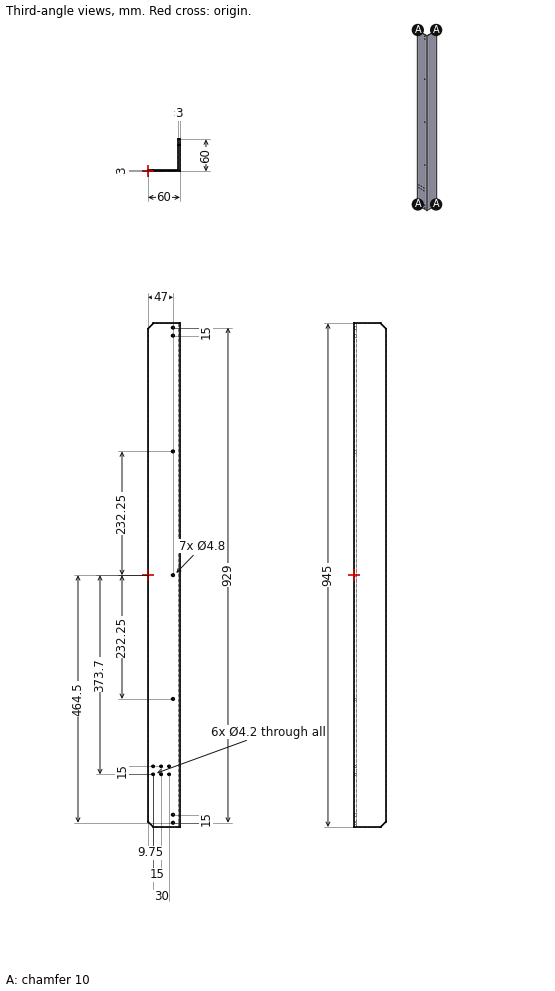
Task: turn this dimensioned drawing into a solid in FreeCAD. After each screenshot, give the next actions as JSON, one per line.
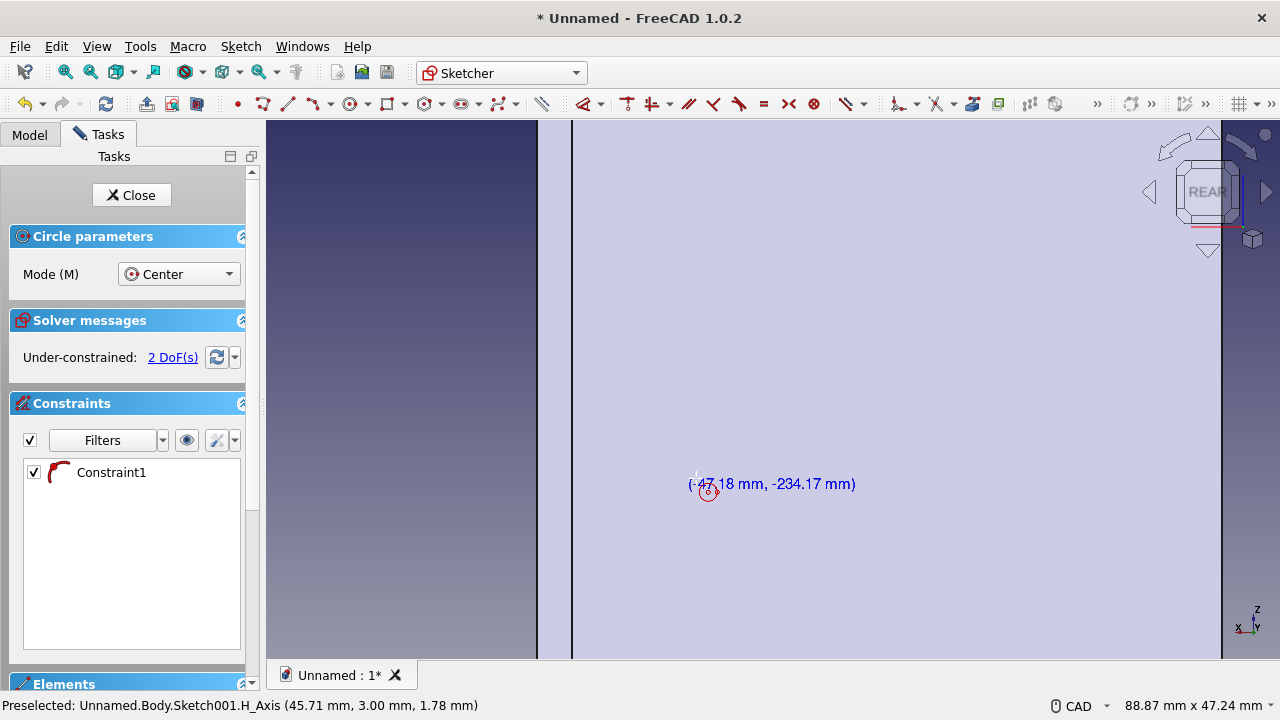
{"action": "scroll", "coordinate": [696, 478], "scroll_direction": "down", "scroll_amount": 17}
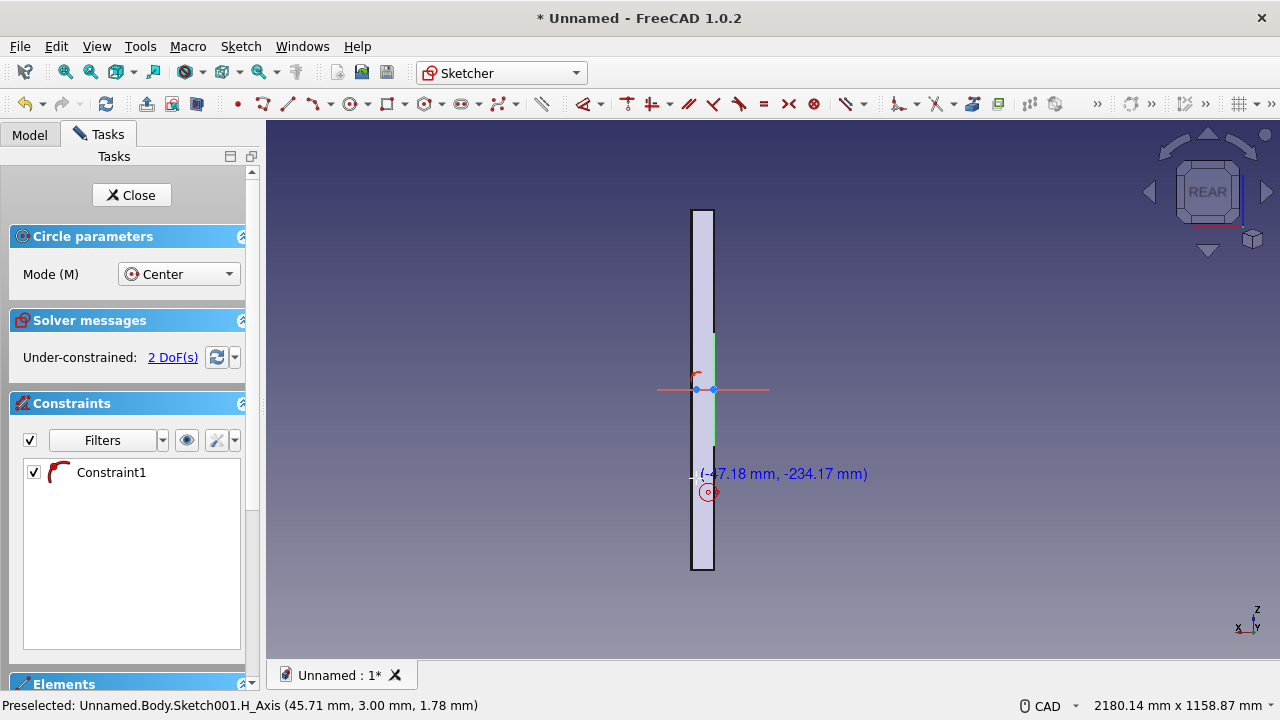
{"action": "left_click", "coordinate": [696, 478]}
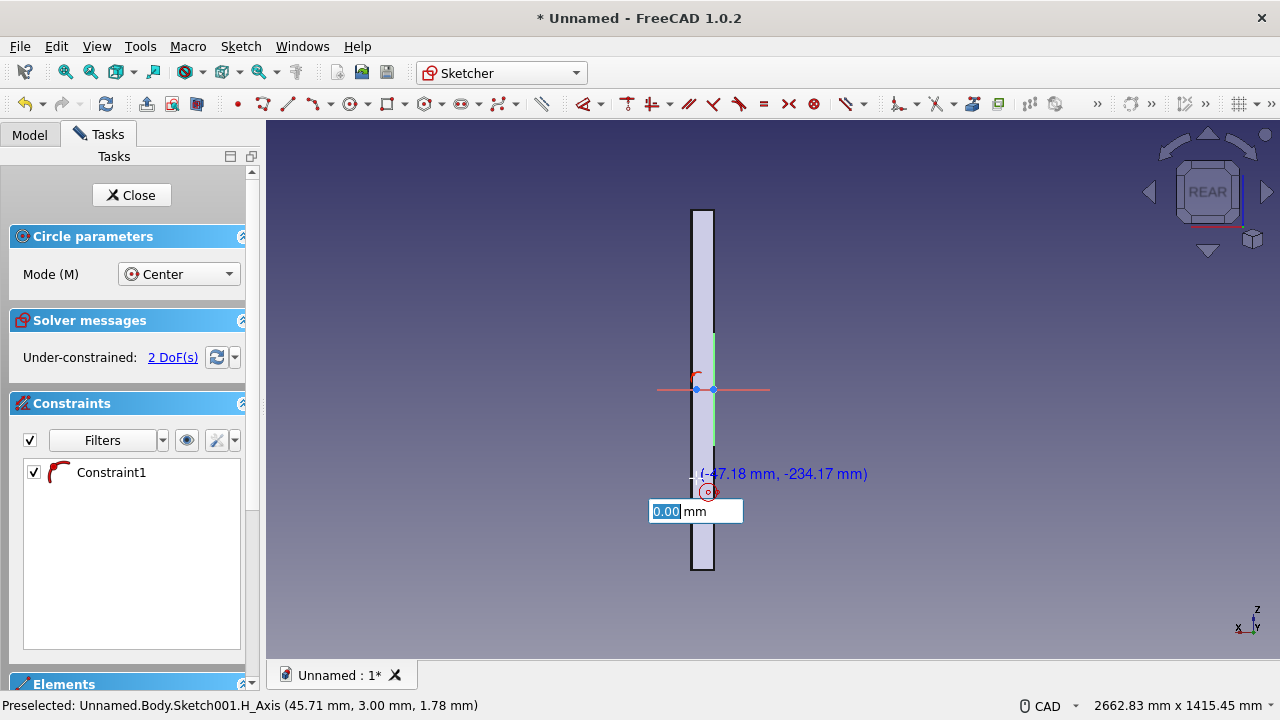
{"action": "scroll", "coordinate": [697, 478], "scroll_direction": "up", "scroll_amount": 15}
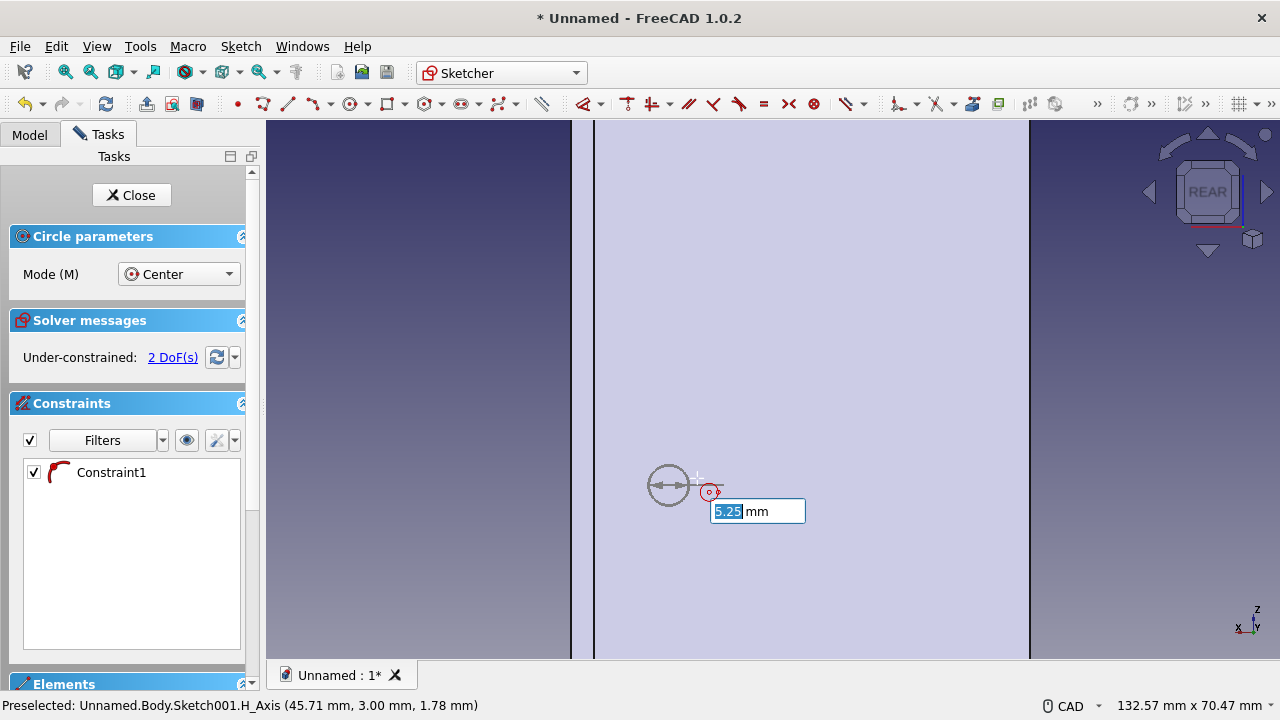
{"action": "left_click", "coordinate": [683, 458]}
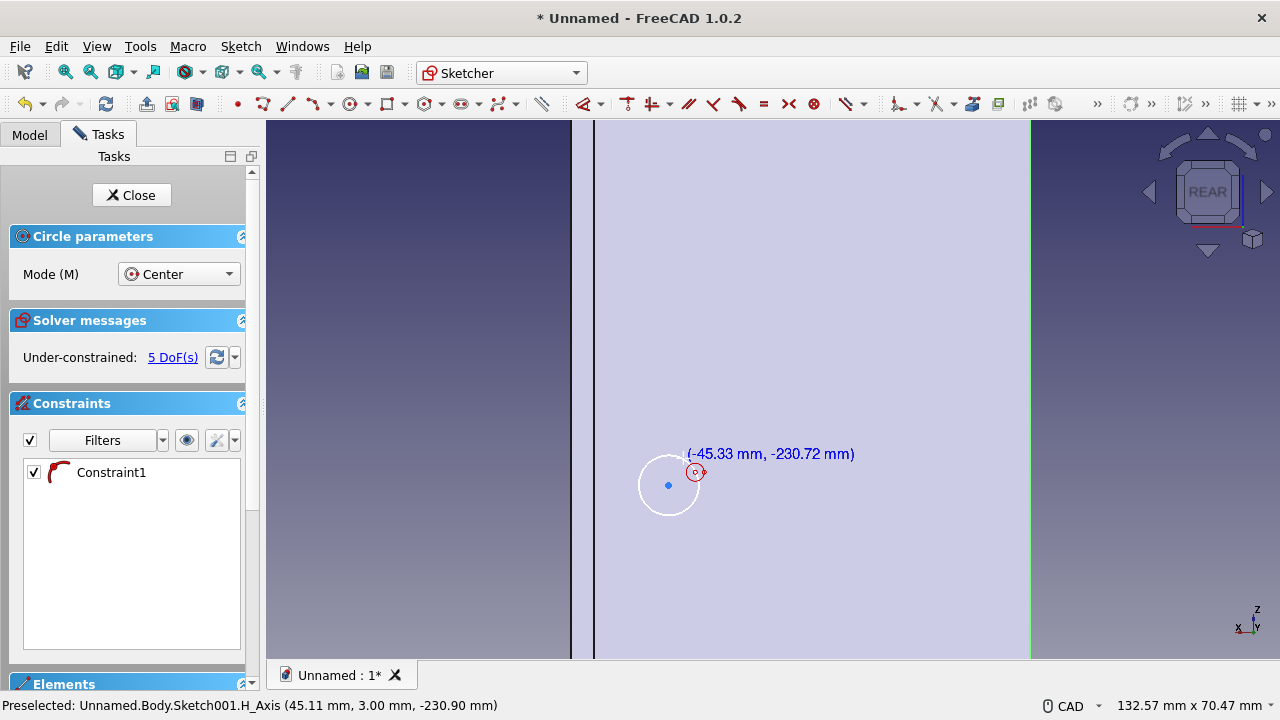
{"action": "scroll", "coordinate": [697, 478], "scroll_direction": "down", "scroll_amount": 15}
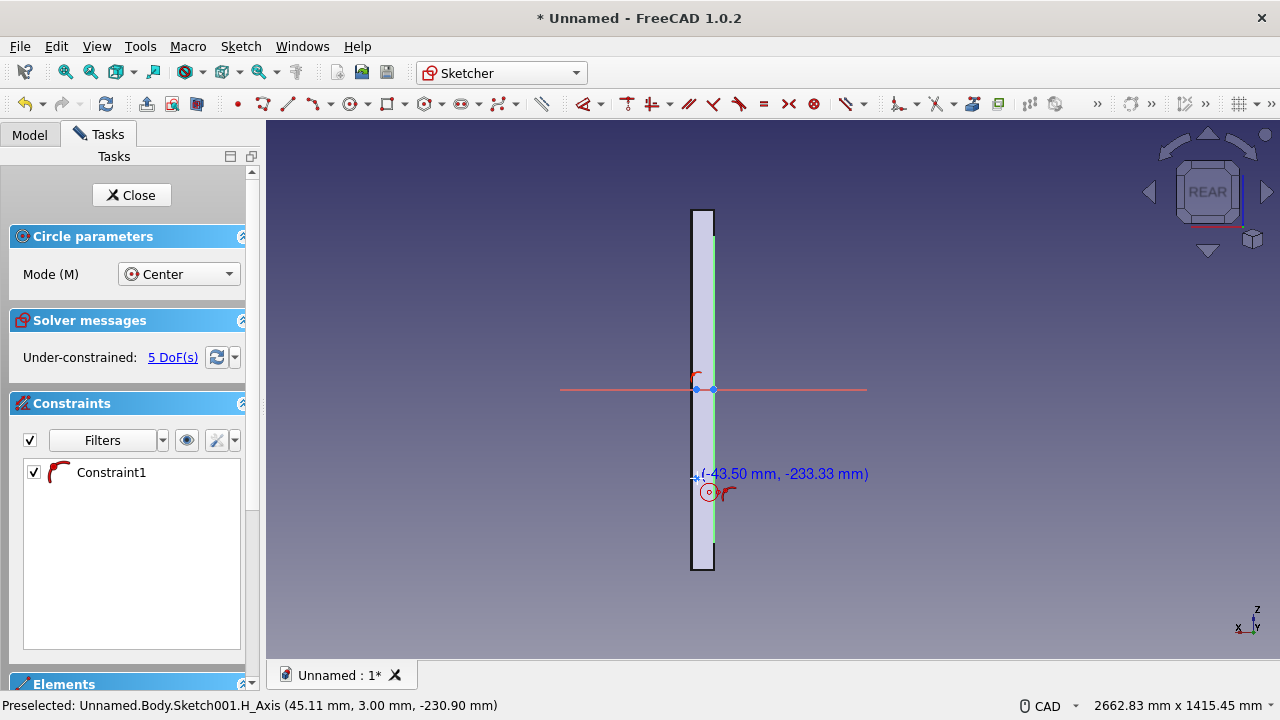
{"action": "scroll", "coordinate": [696, 567], "scroll_direction": "up", "scroll_amount": 17}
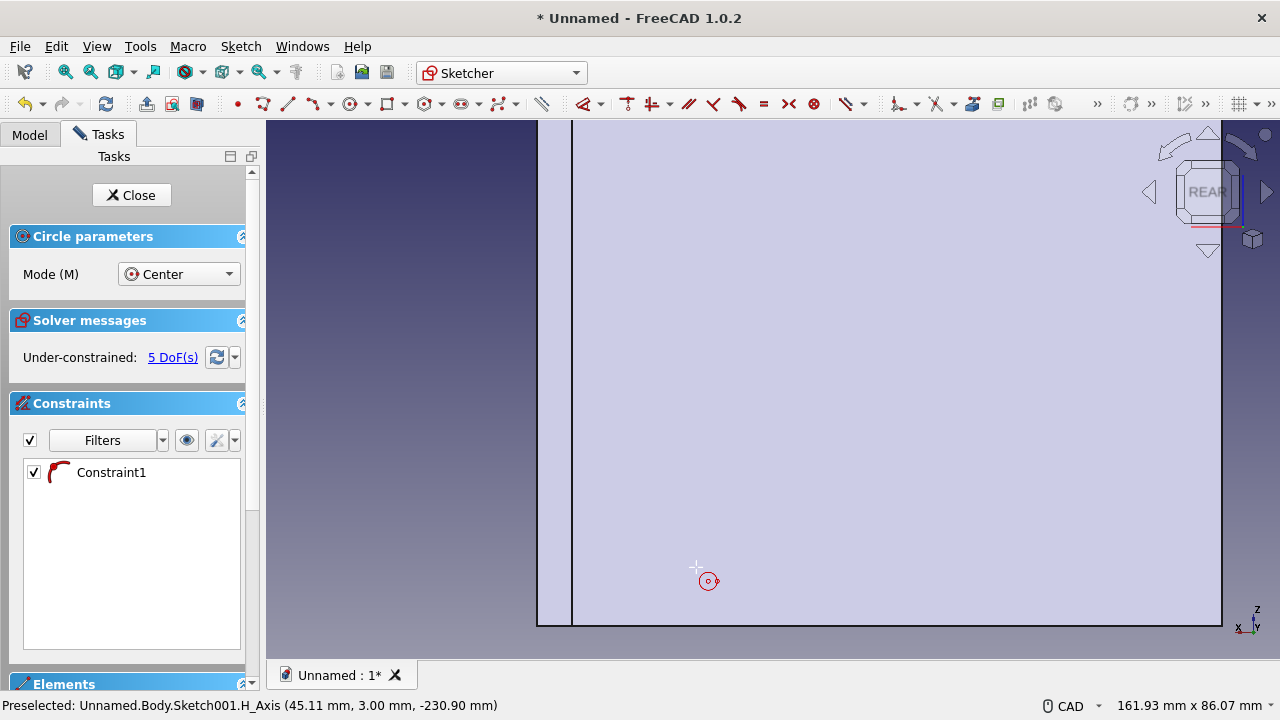
{"action": "scroll", "coordinate": [696, 567], "scroll_direction": "down", "scroll_amount": 17}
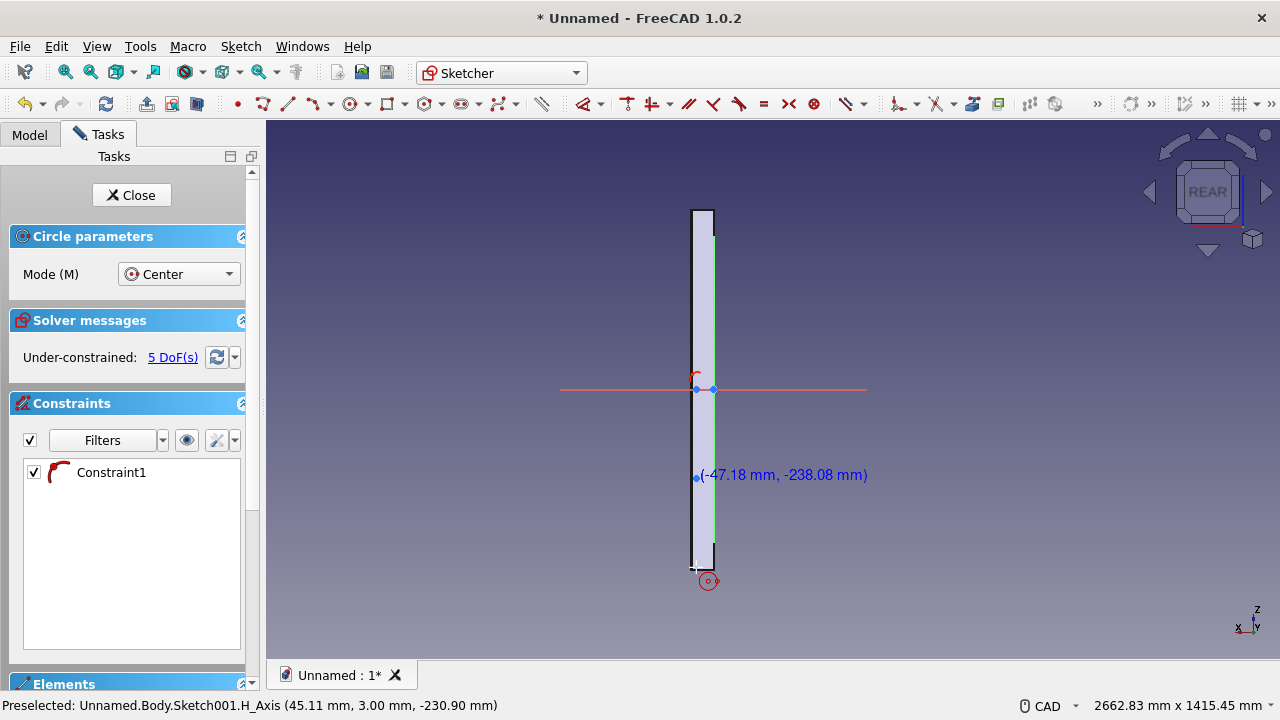
{"action": "left_click", "coordinate": [696, 567]}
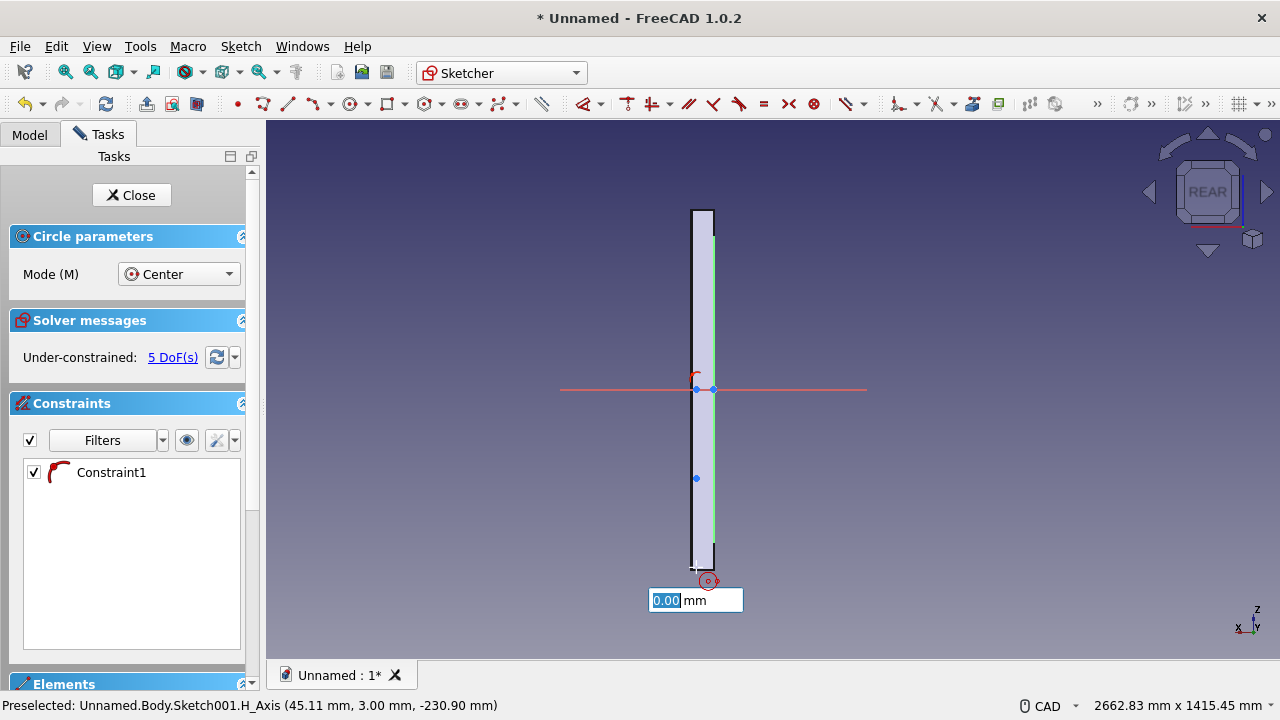
{"action": "scroll", "coordinate": [697, 566], "scroll_direction": "up", "scroll_amount": 15}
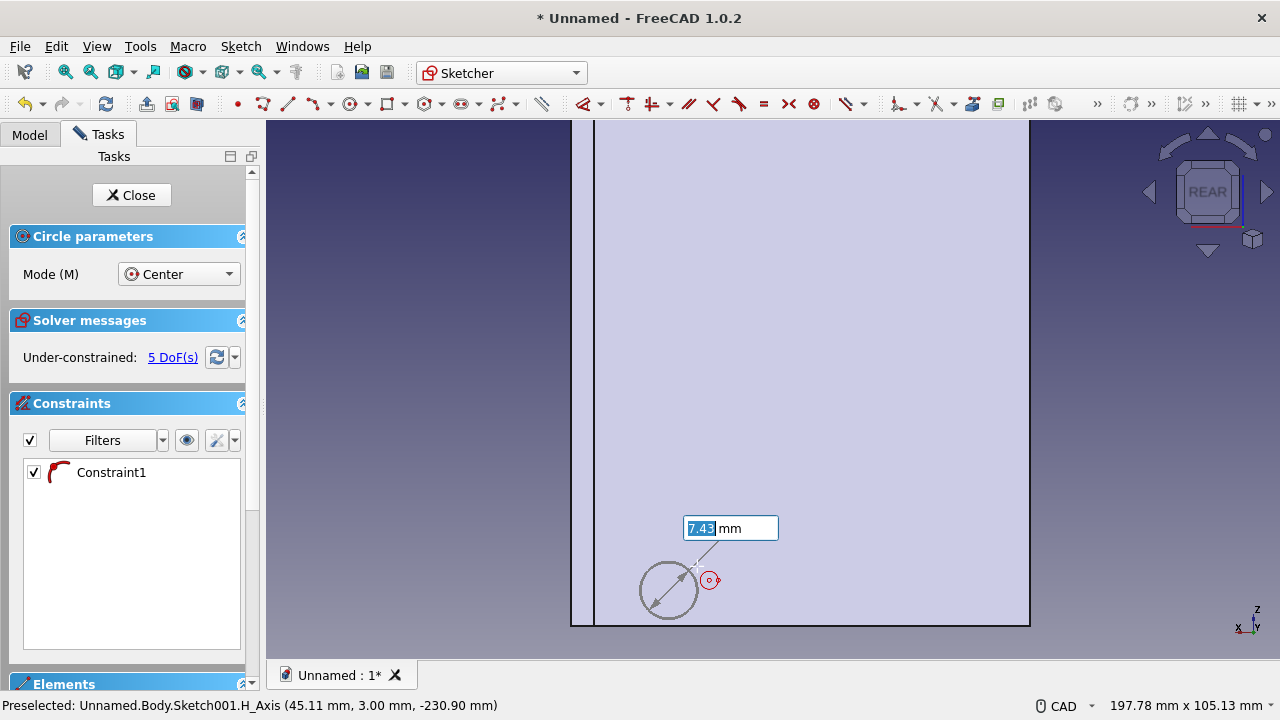
{"action": "left_click", "coordinate": [683, 551]}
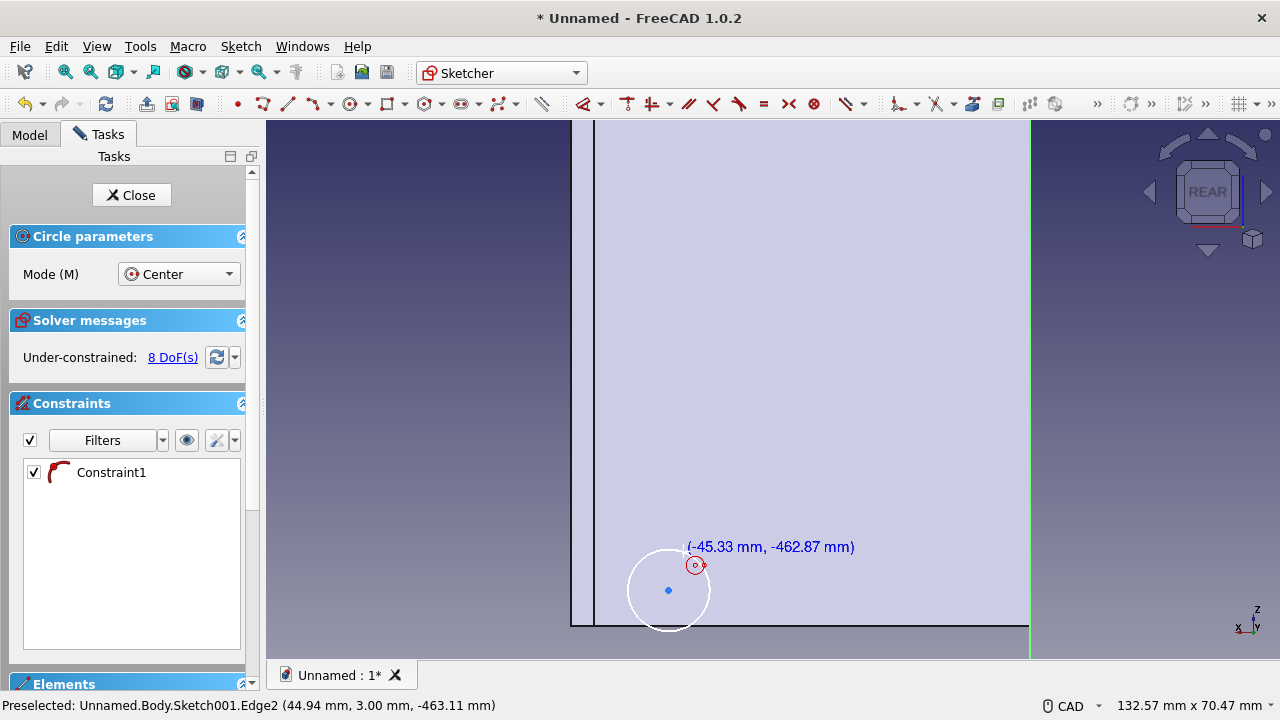
{"action": "scroll", "coordinate": [697, 566], "scroll_direction": "down", "scroll_amount": 15}